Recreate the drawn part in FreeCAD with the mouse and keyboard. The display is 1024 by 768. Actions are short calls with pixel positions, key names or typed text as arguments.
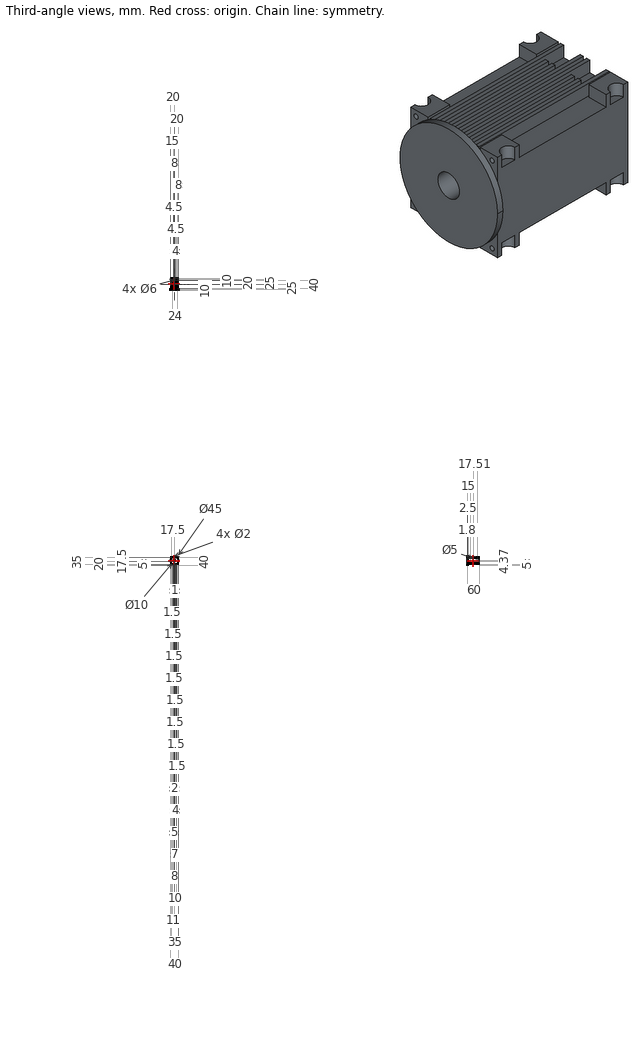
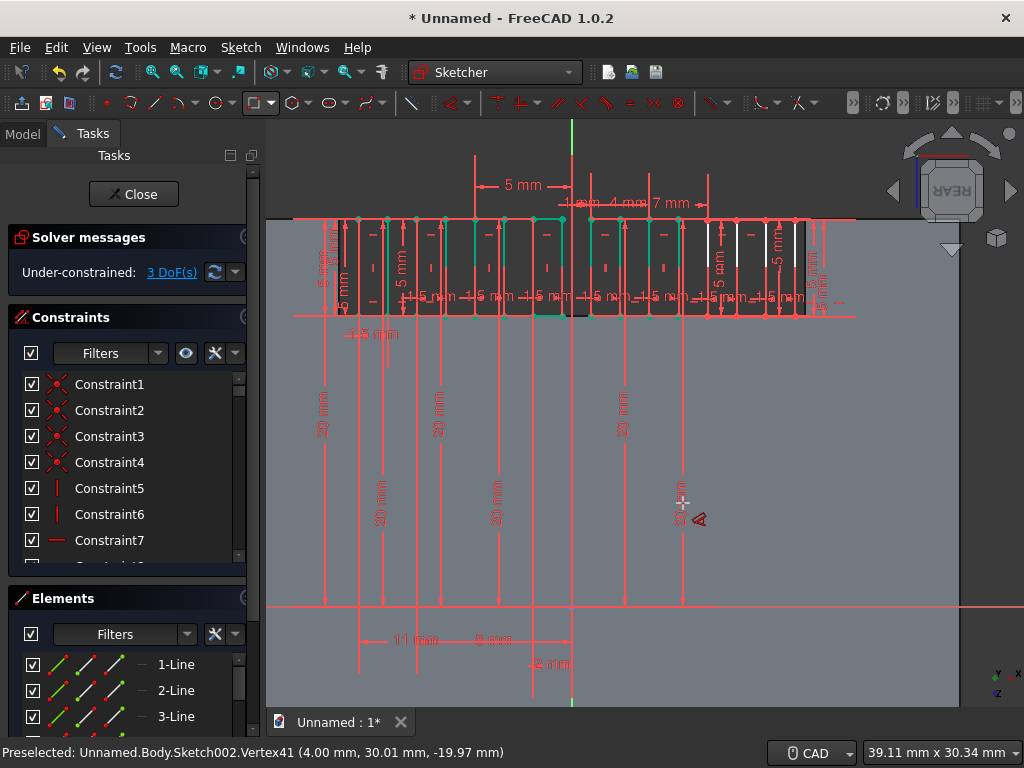
click(708, 220)
click(742, 414)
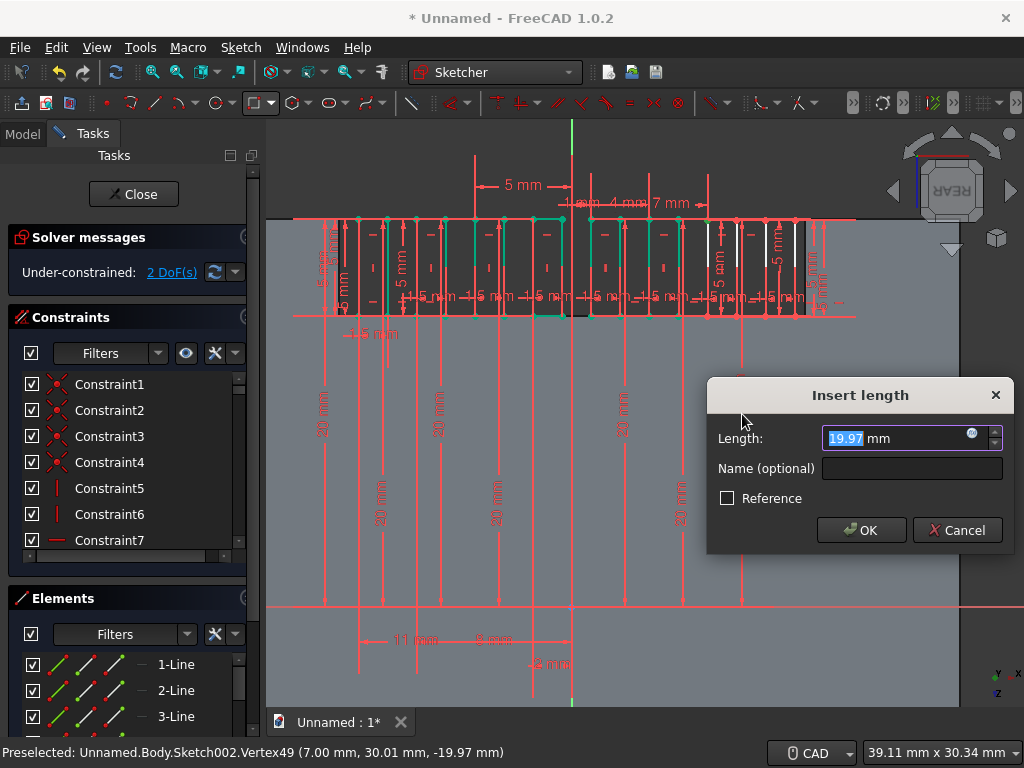
text(20)
key(Return)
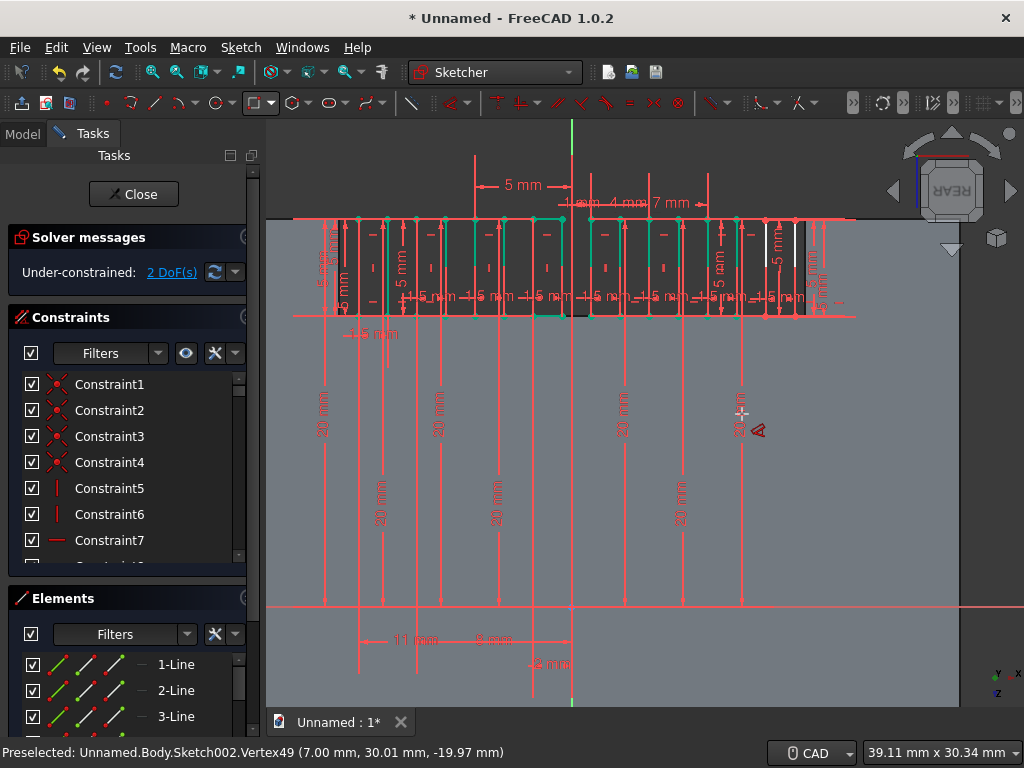
click(766, 220)
click(669, 641)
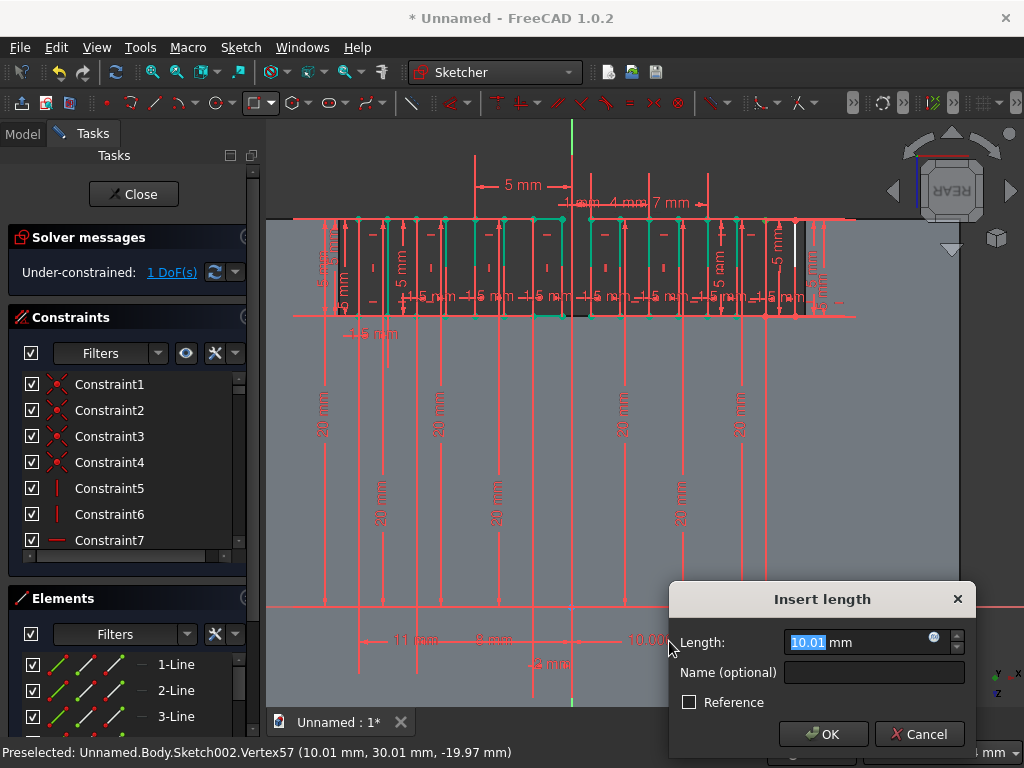
text(10)
key(Return)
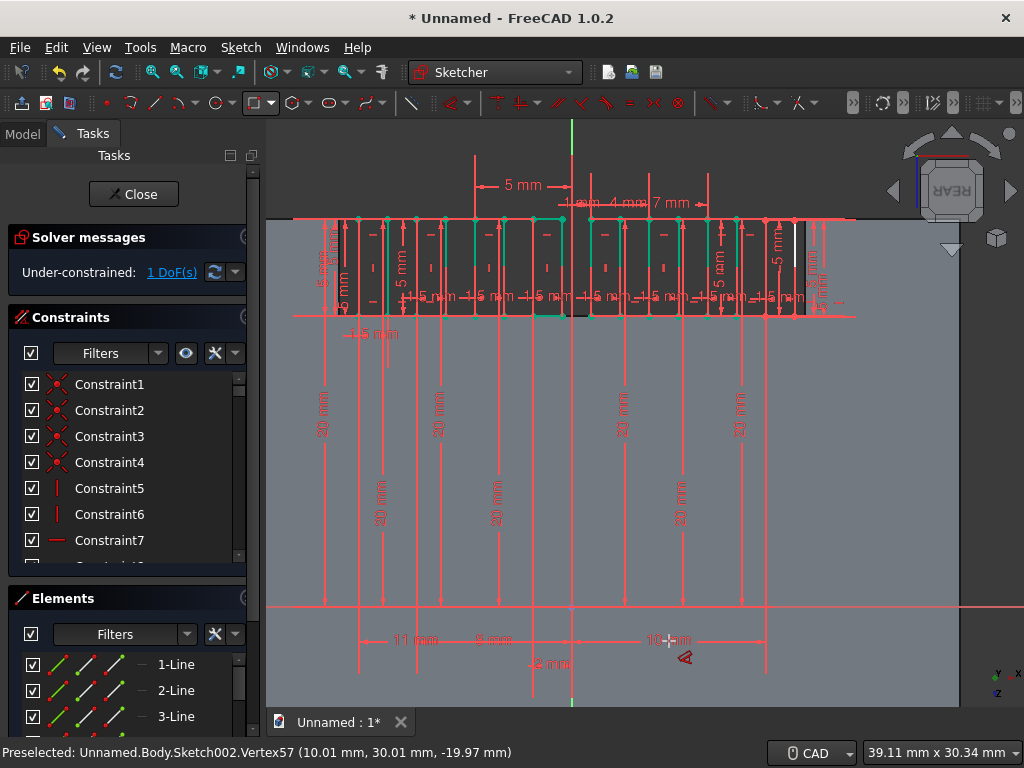
click(766, 220)
click(800, 503)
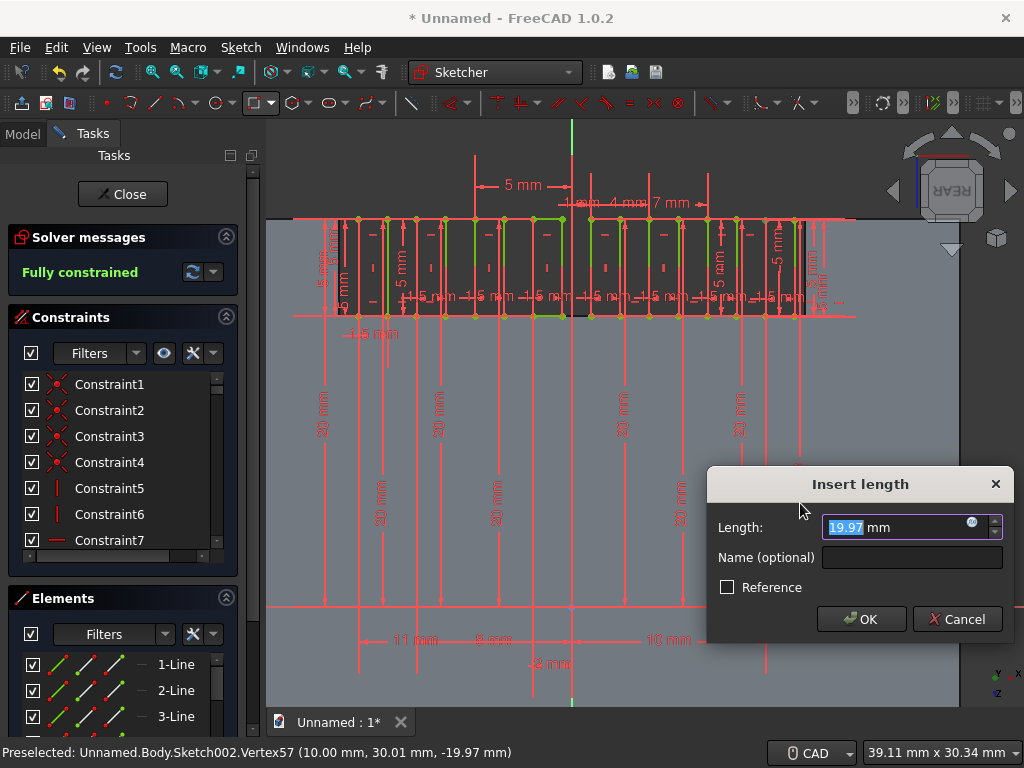
text(20)
key(Return)
key(Escape)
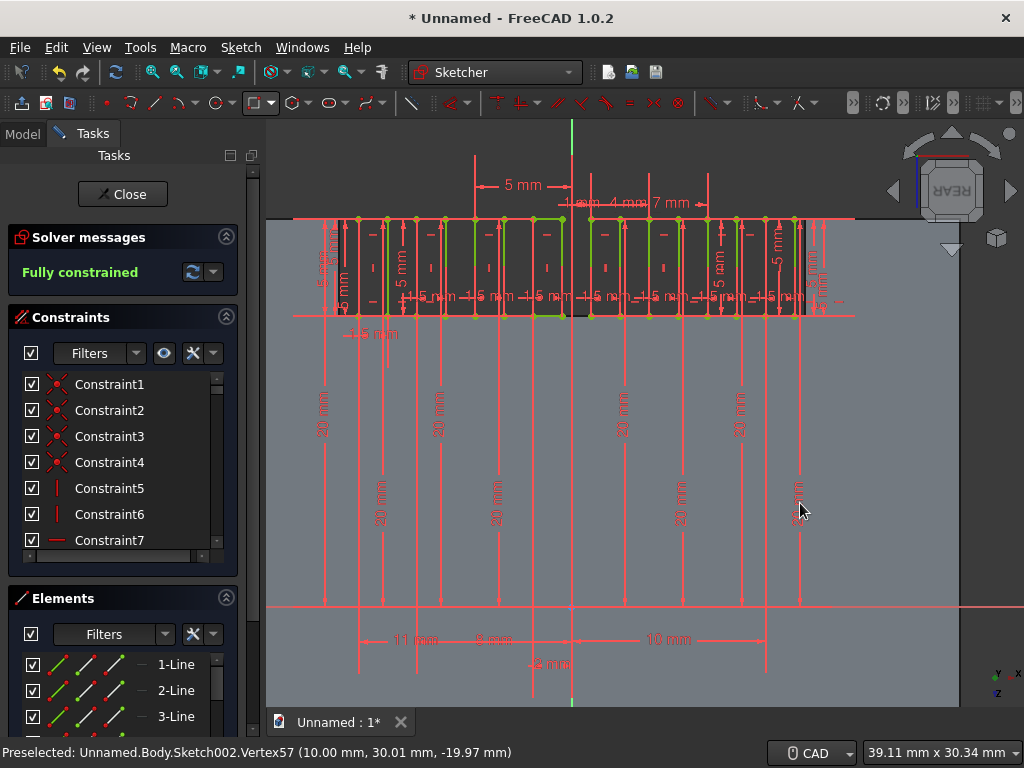
click(123, 194)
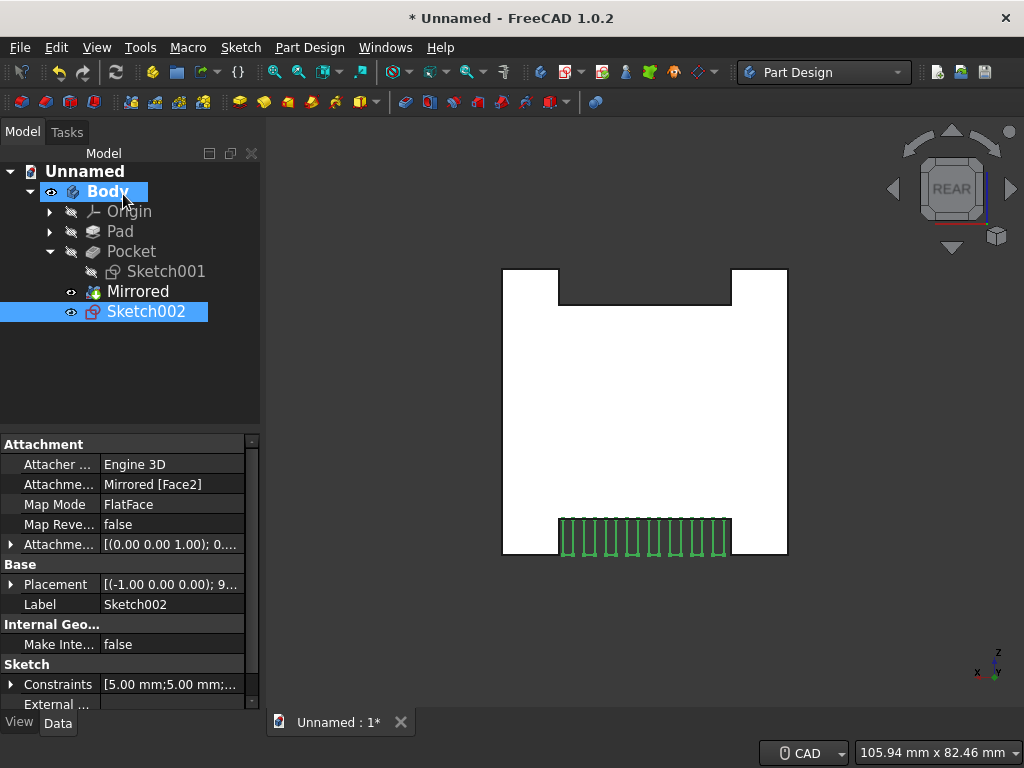
click(240, 102)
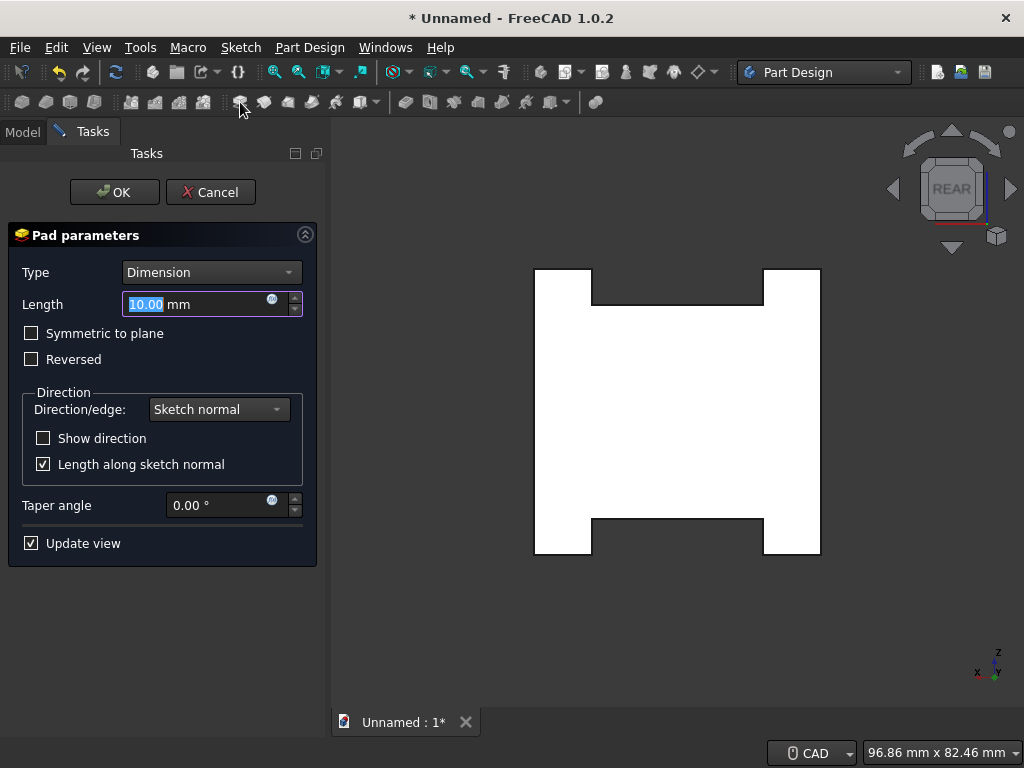
text(60)
key(Tab)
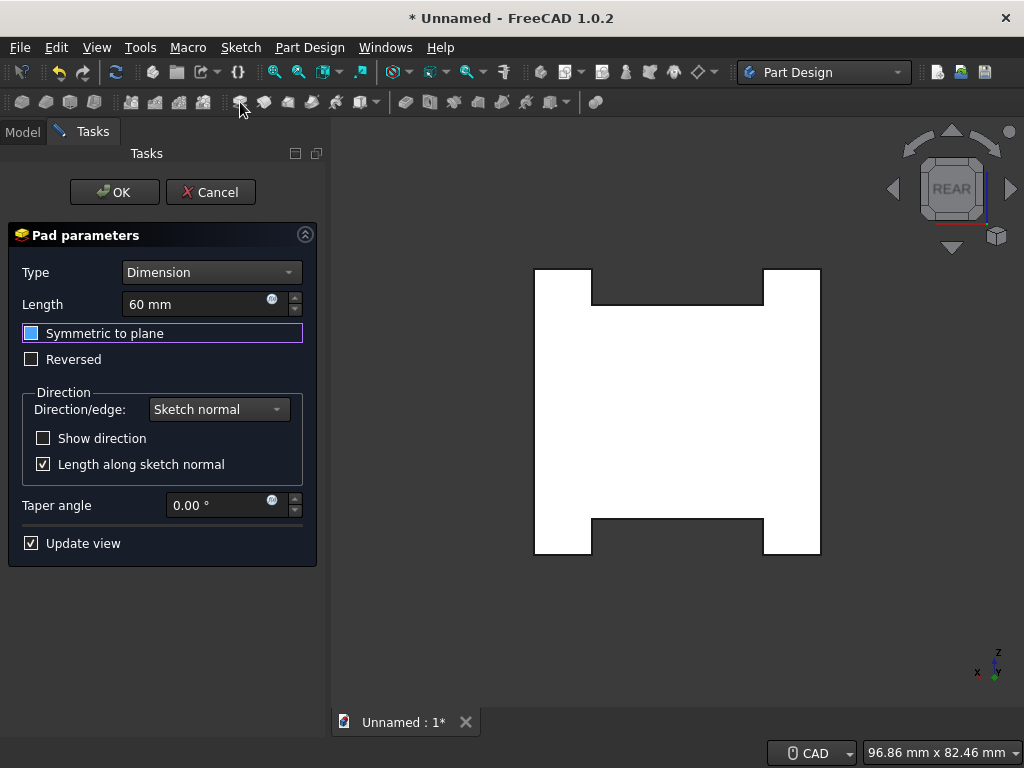
click(30, 359)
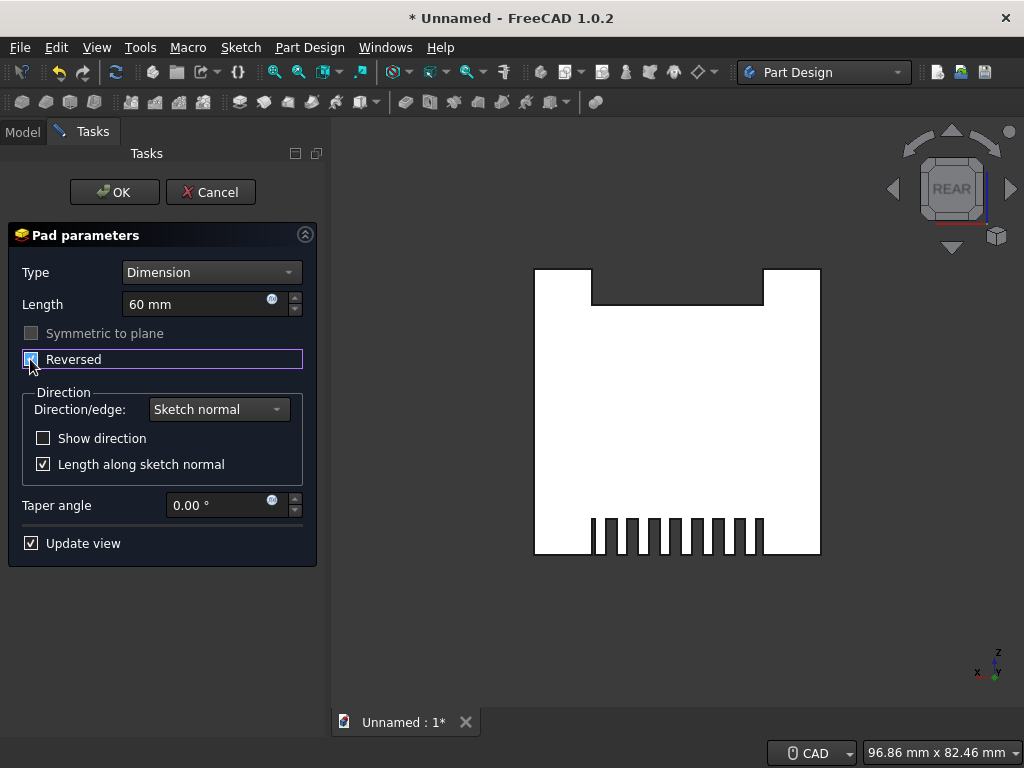
click(115, 192)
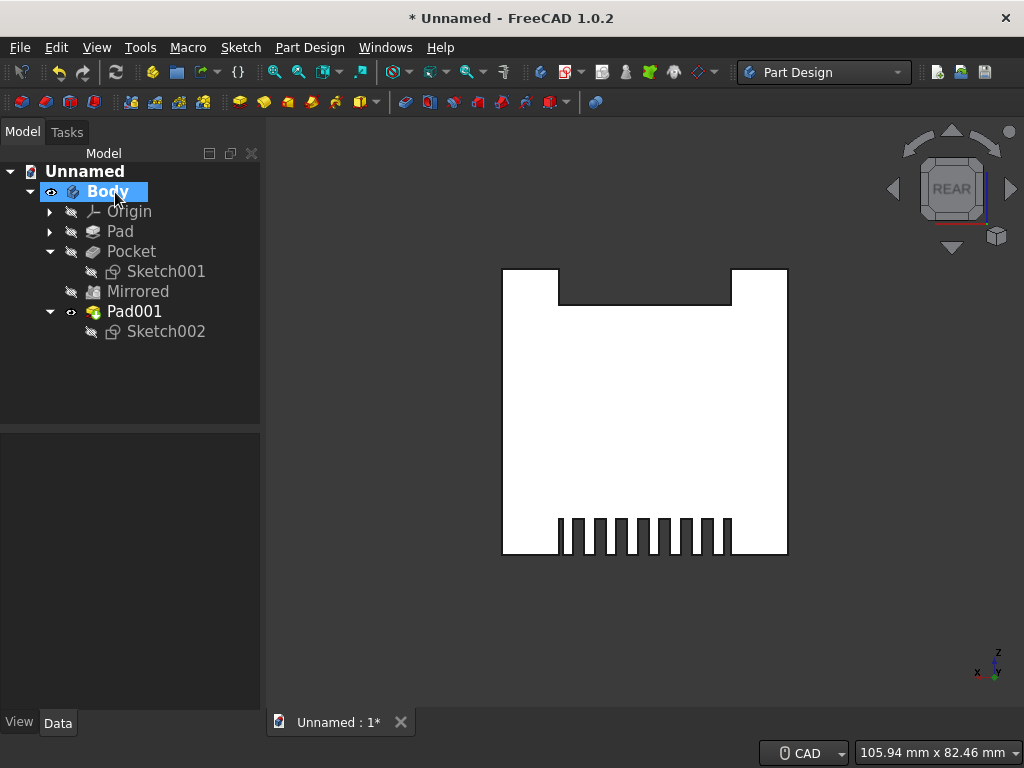
key(5)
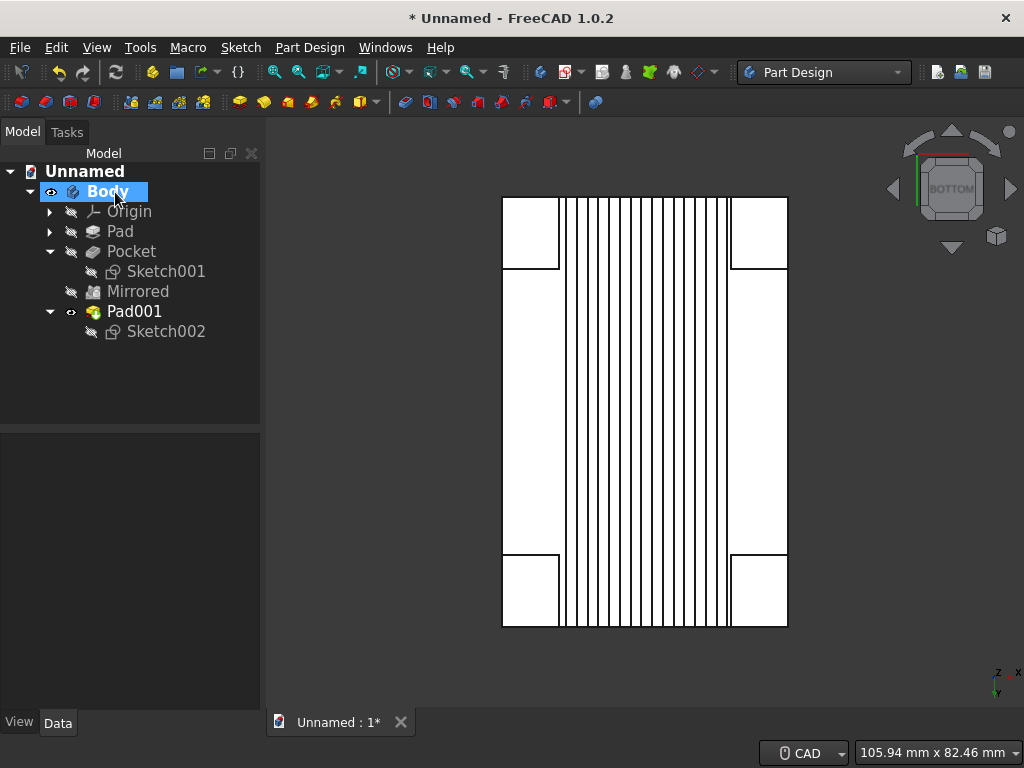
scroll(658, 595, up, 5)